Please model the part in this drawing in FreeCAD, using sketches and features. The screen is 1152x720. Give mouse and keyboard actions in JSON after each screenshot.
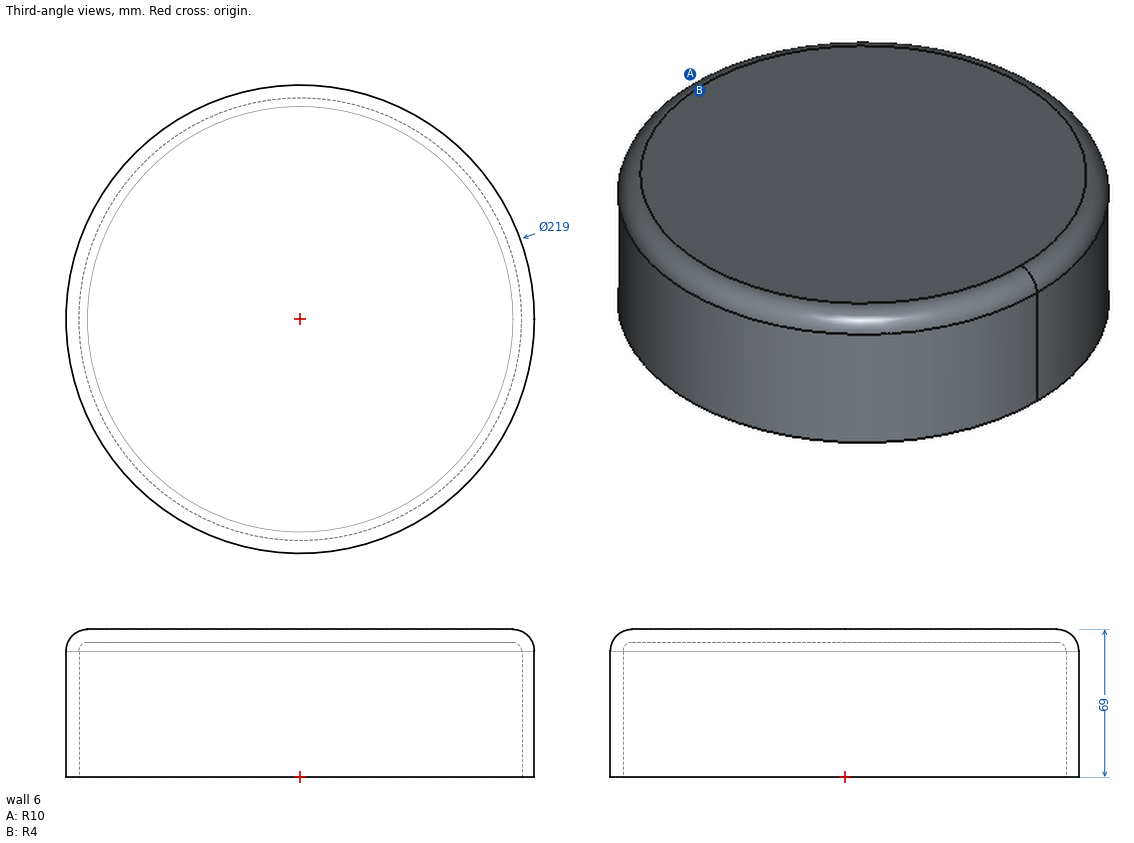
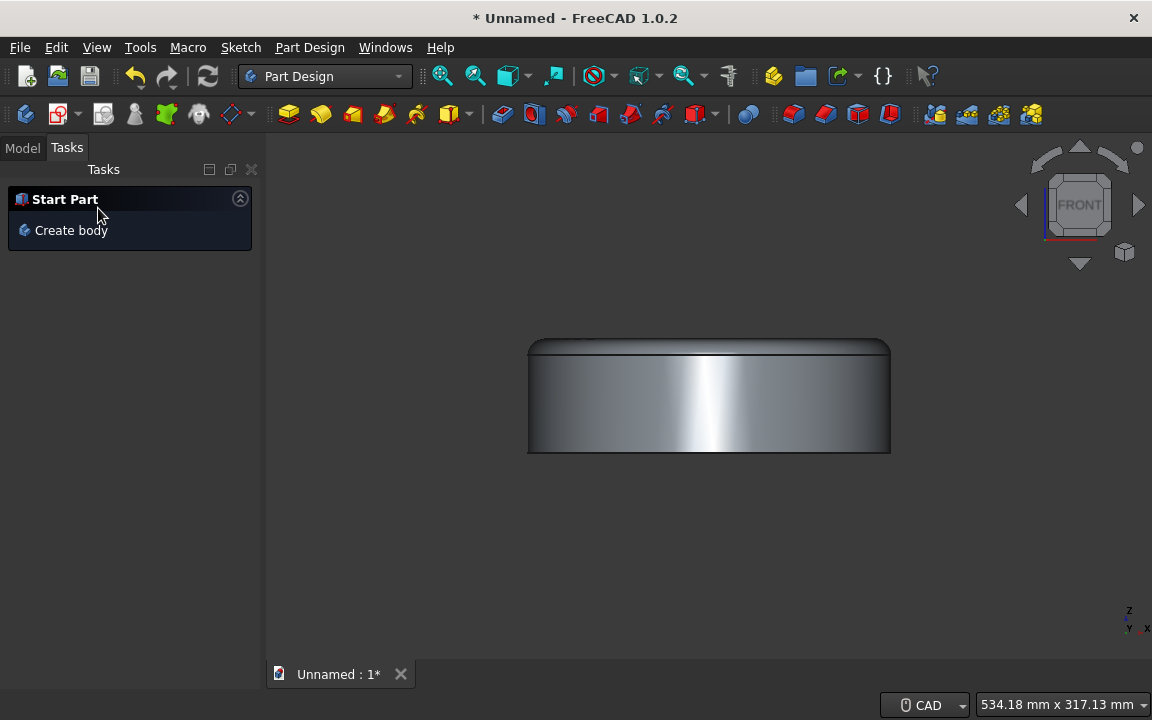
{"action": "key", "text": "v f"}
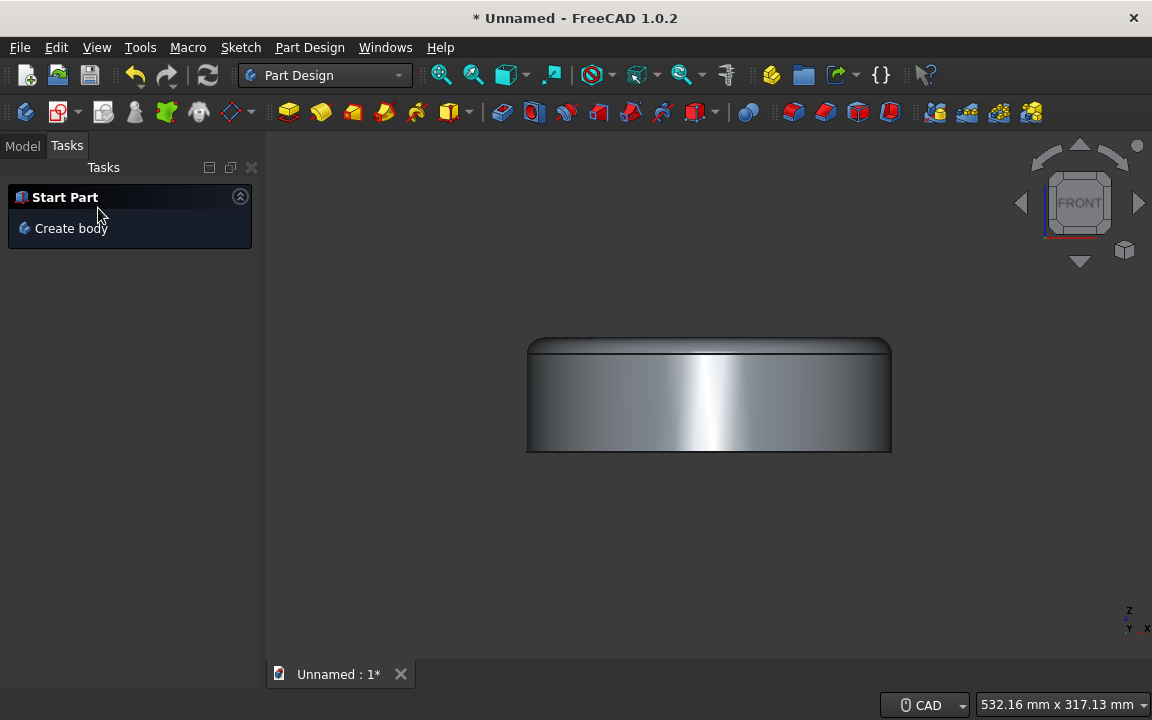
{"action": "key", "text": "3"}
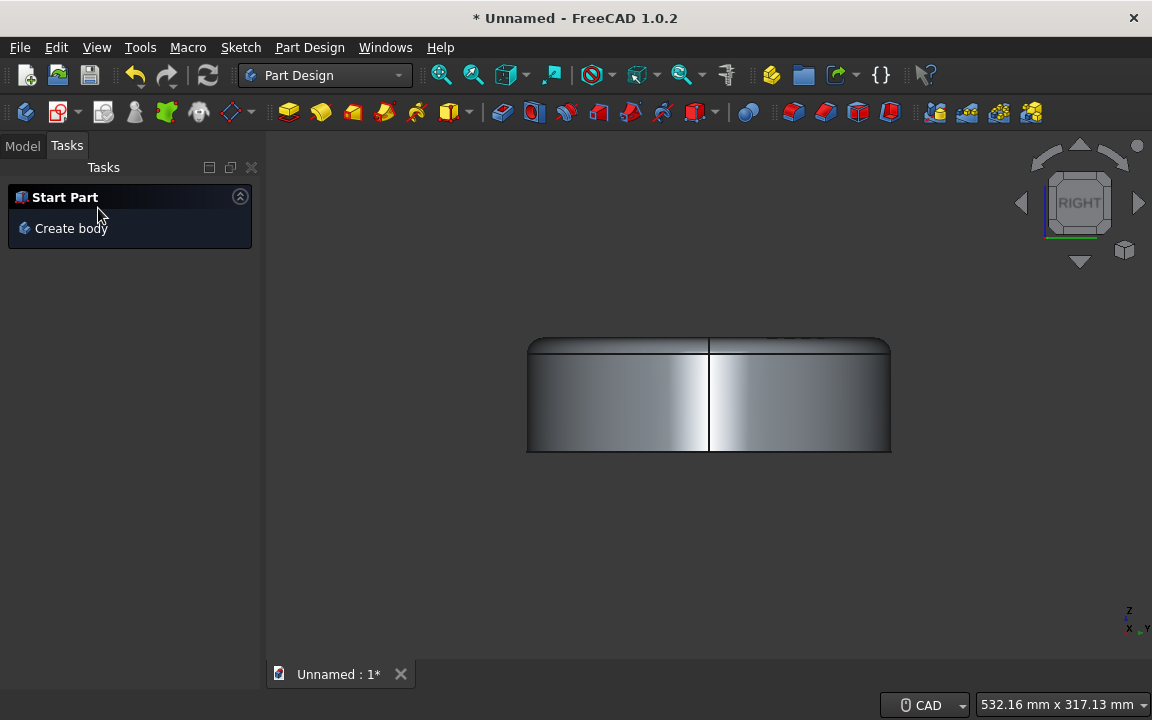
{"action": "key", "text": "v f"}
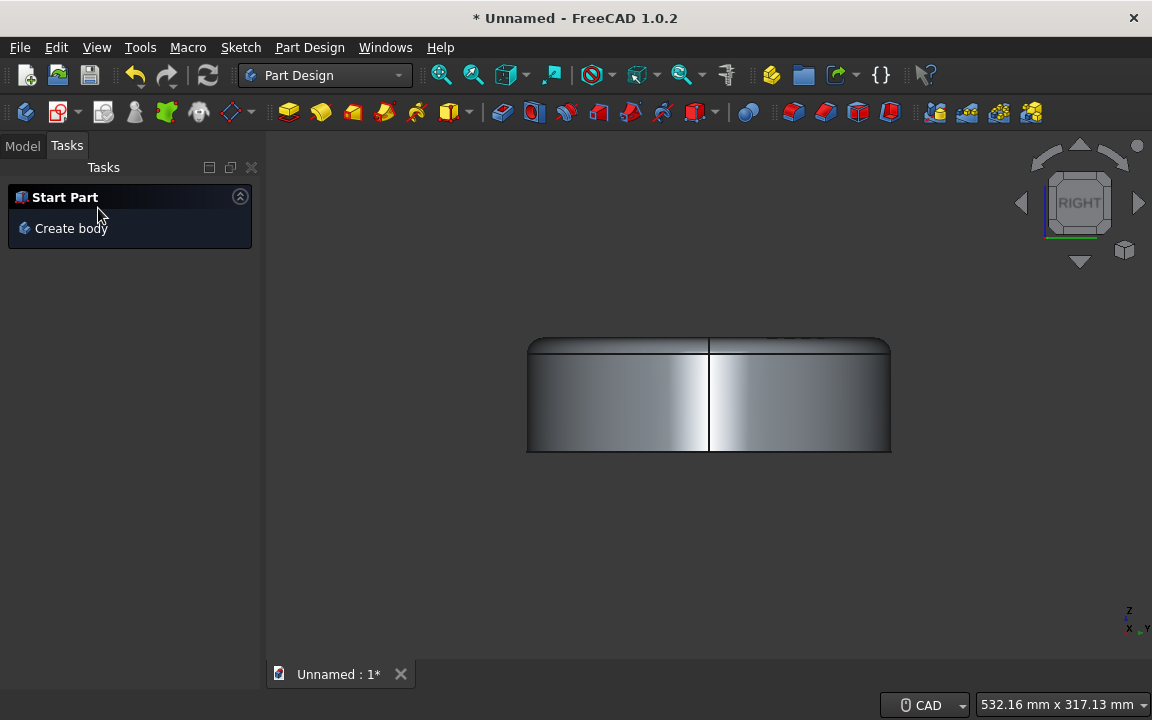
{"action": "key", "text": "5"}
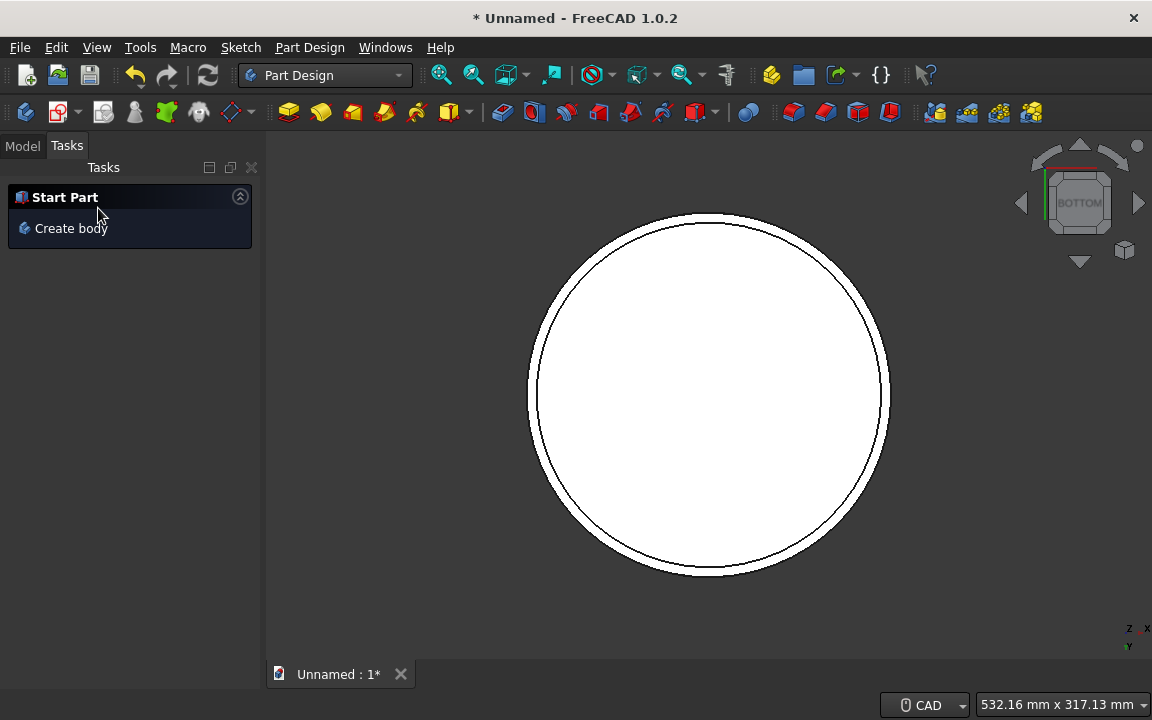
{"action": "key", "text": "4"}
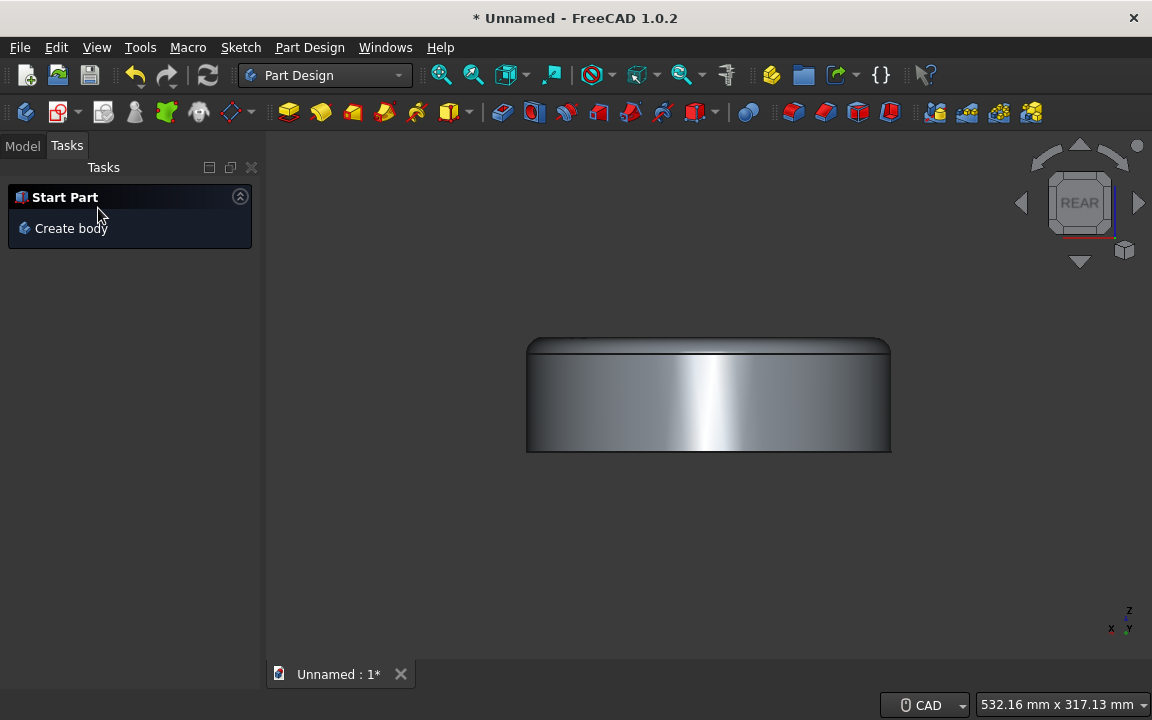
{"action": "key", "text": "v f"}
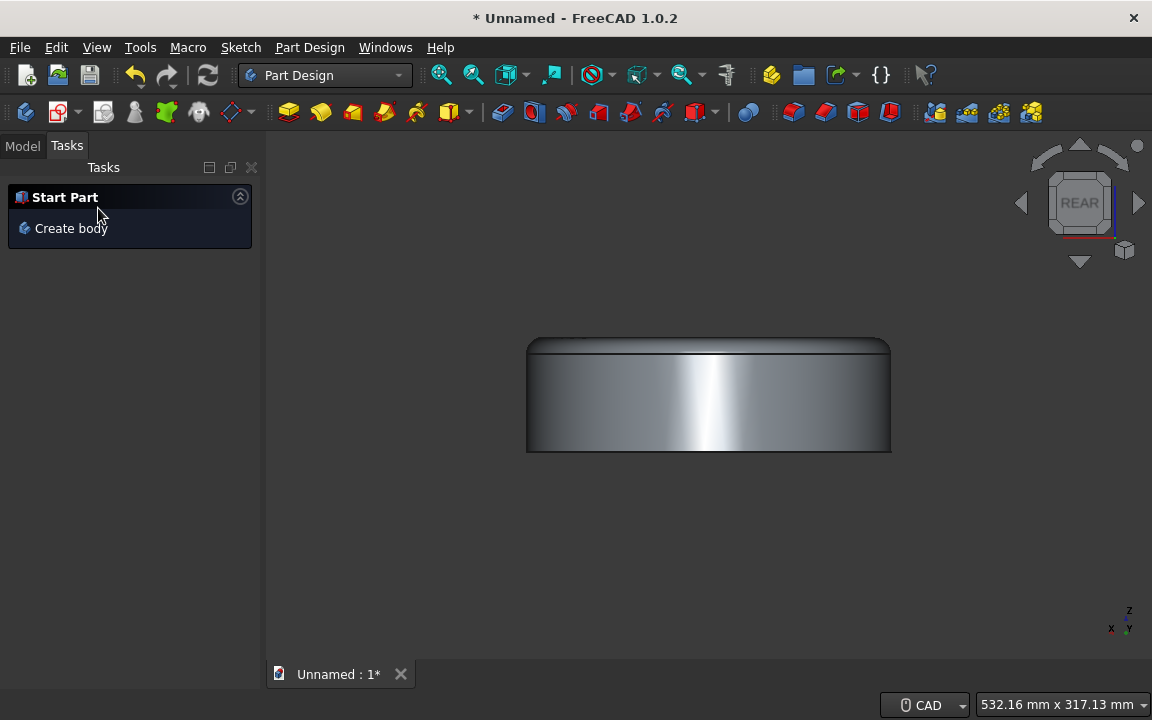
{"action": "key", "text": "6"}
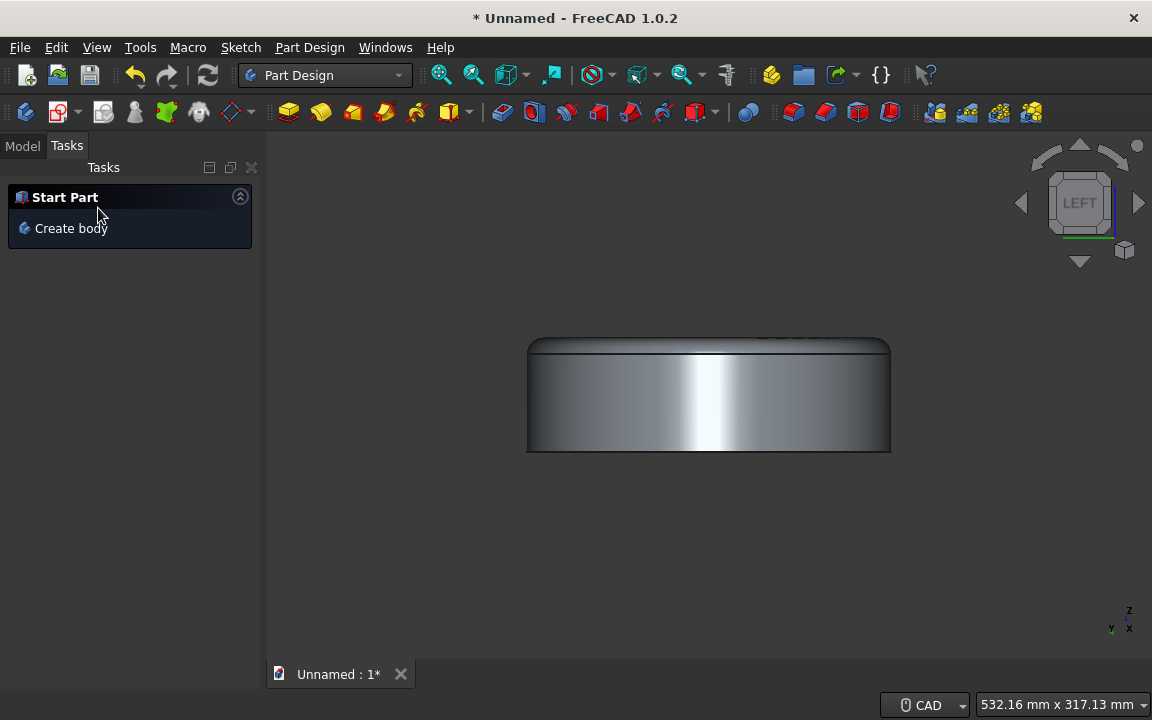
{"action": "key", "text": "v f"}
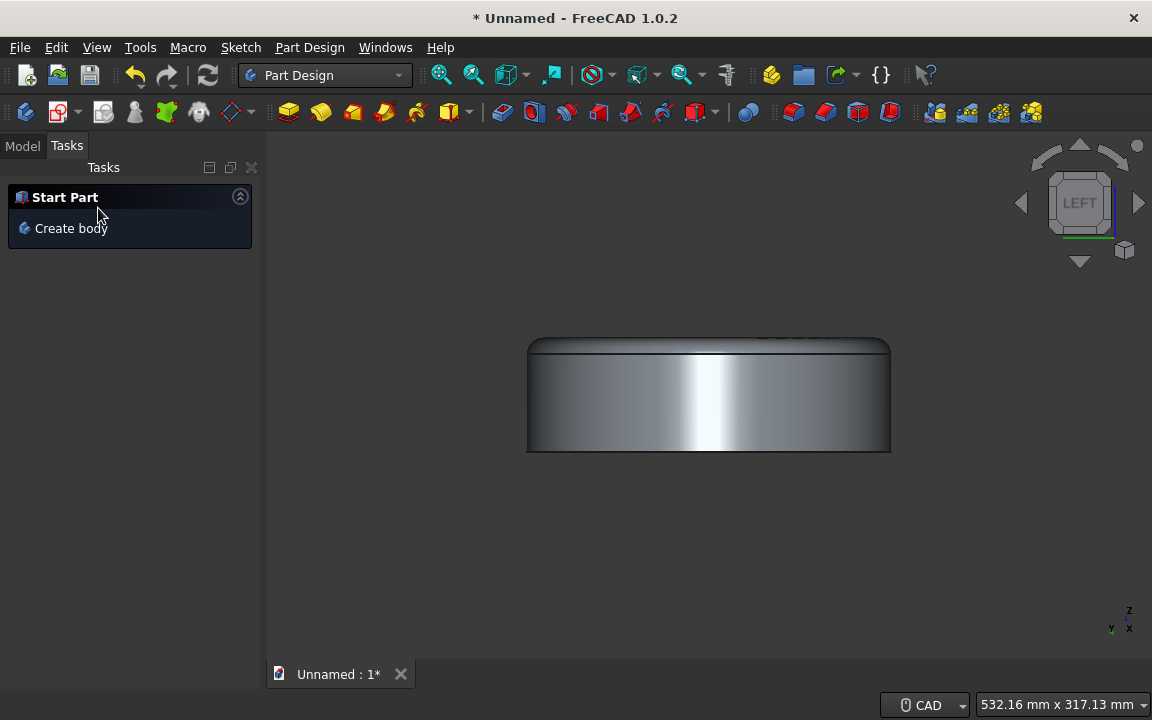
{"action": "key", "text": "v 3"}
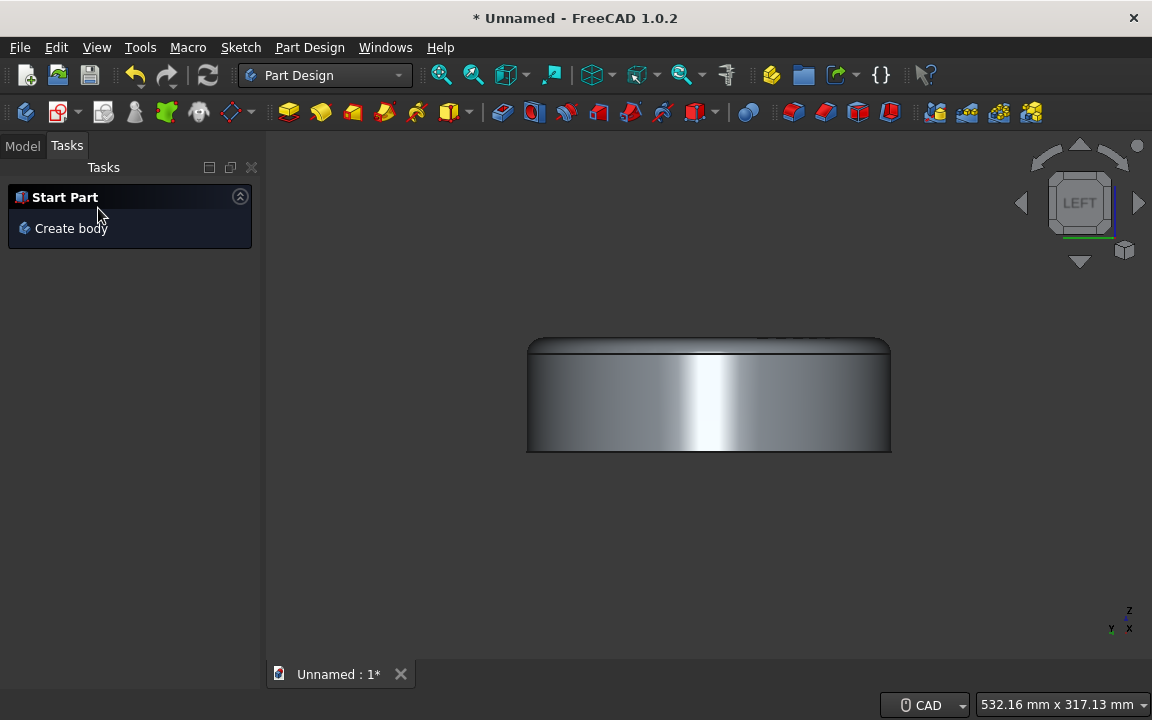
{"action": "key", "text": "0"}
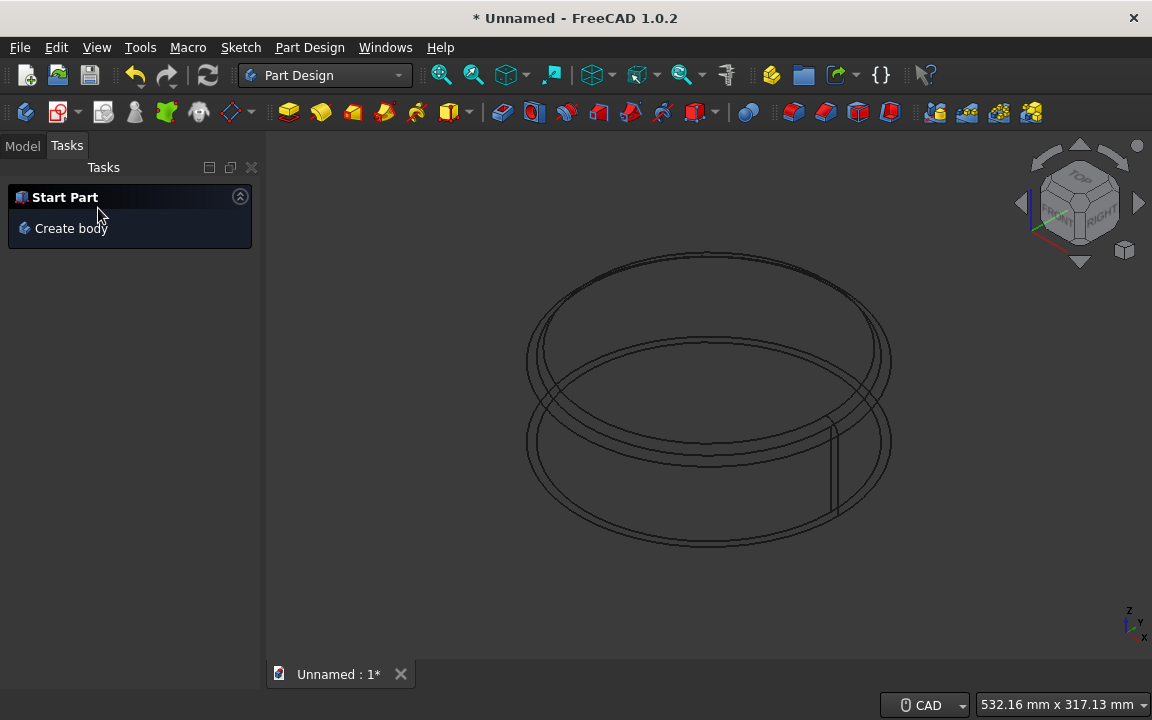
{"action": "left_click", "coordinate": [555, 400]}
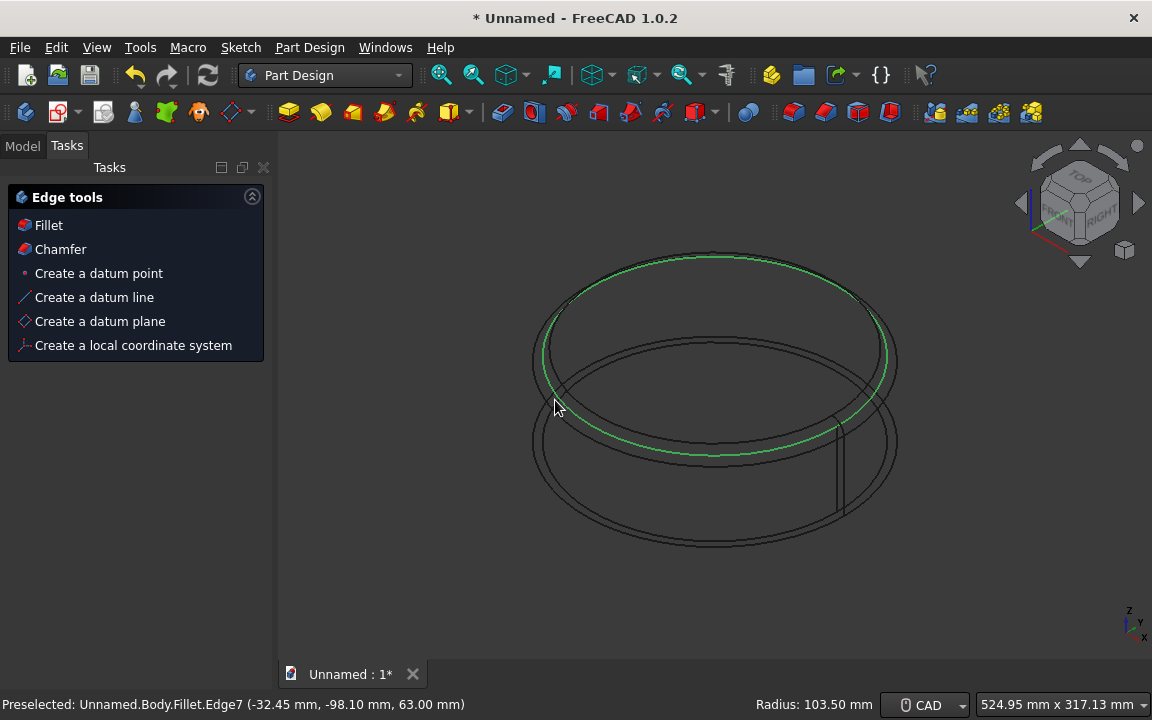
{"action": "key", "text": "v 1"}